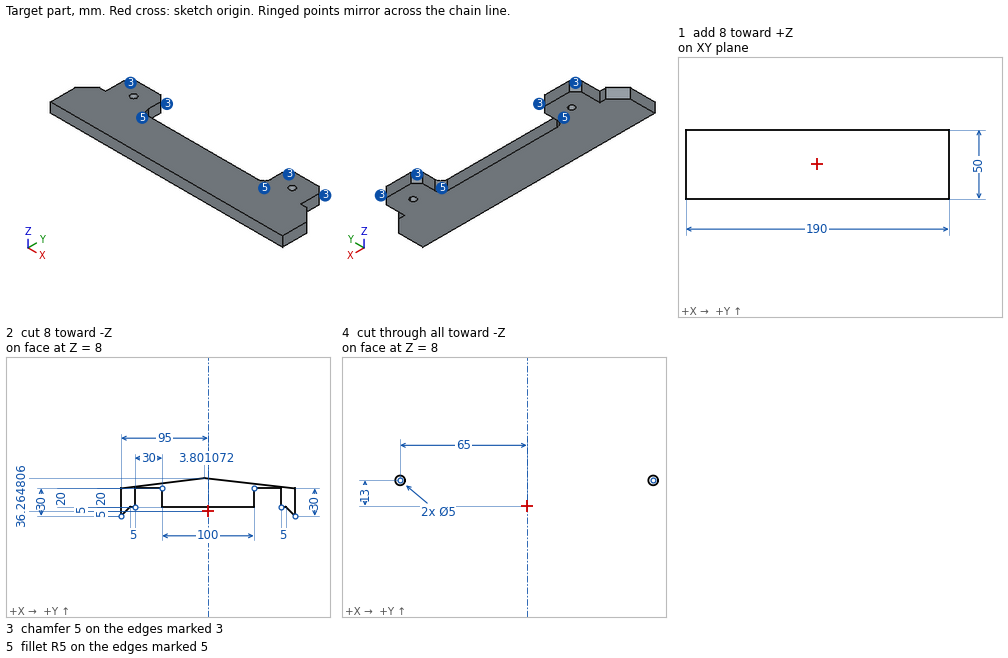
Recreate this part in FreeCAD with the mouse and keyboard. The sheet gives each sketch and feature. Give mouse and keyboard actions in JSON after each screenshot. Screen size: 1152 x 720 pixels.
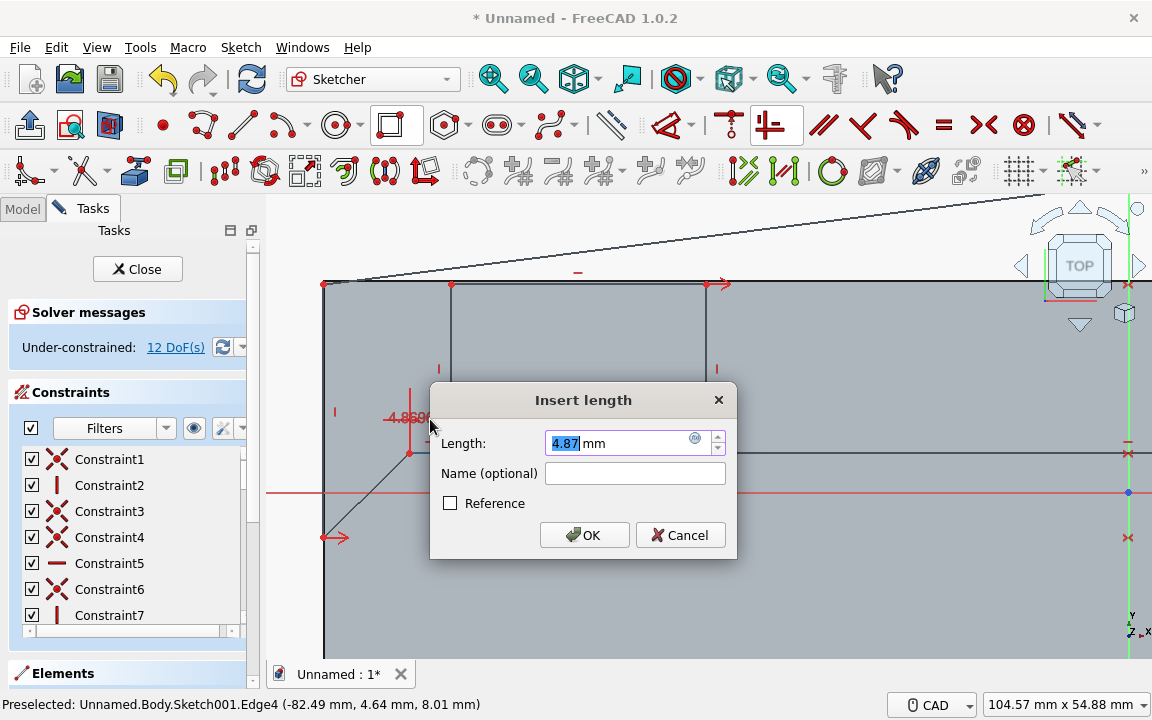
{"action": "type", "text": "5"}
{"action": "key", "text": "Return"}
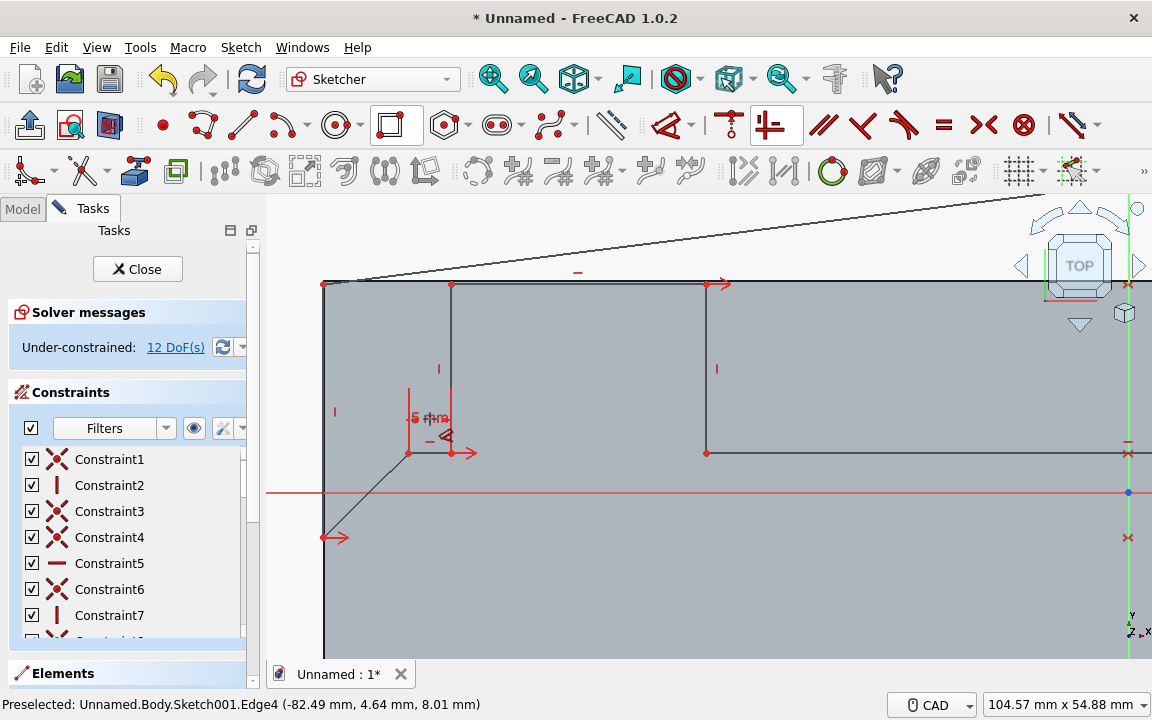
{"action": "scroll", "coordinate": [430, 455], "scroll_direction": "down", "scroll_amount": 6}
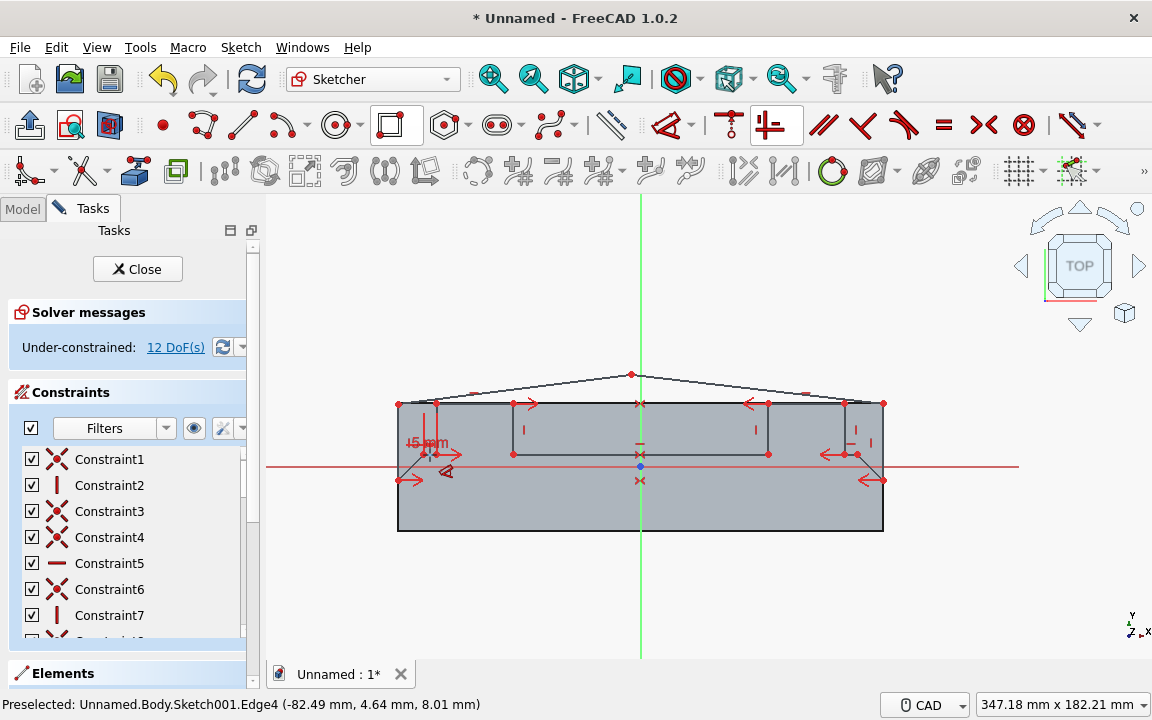
{"action": "scroll", "coordinate": [849, 455], "scroll_direction": "up", "scroll_amount": 7}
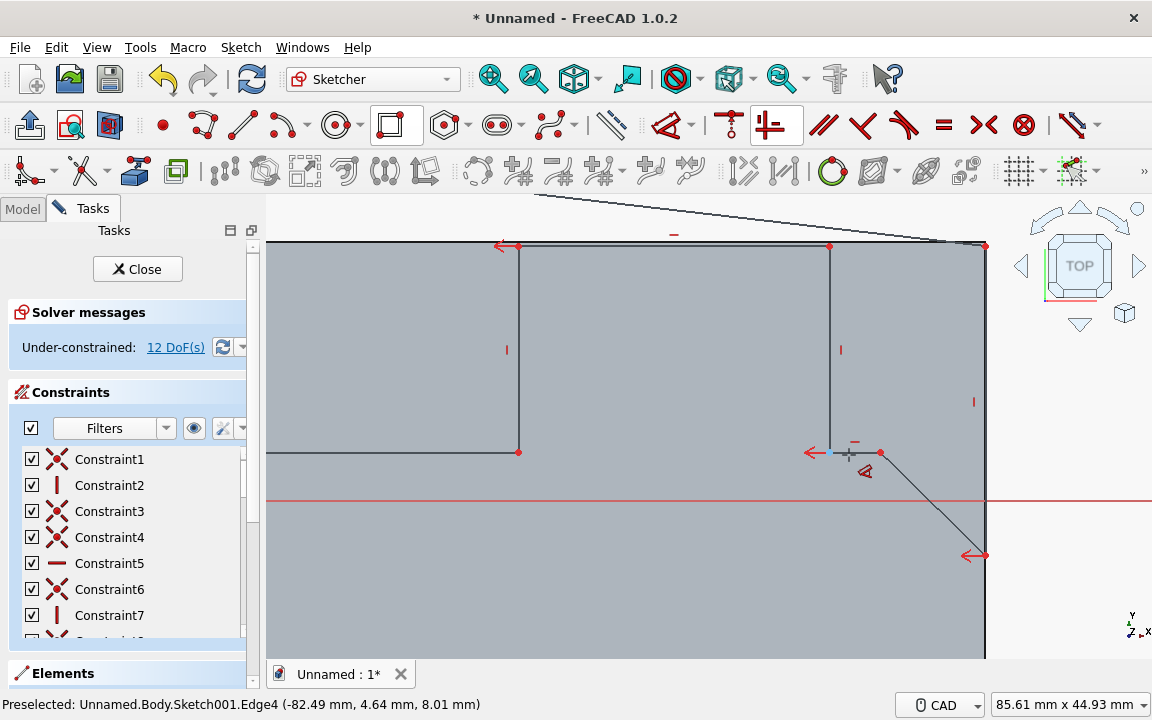
{"action": "left_click", "coordinate": [845, 453]}
{"action": "left_click", "coordinate": [855, 487]}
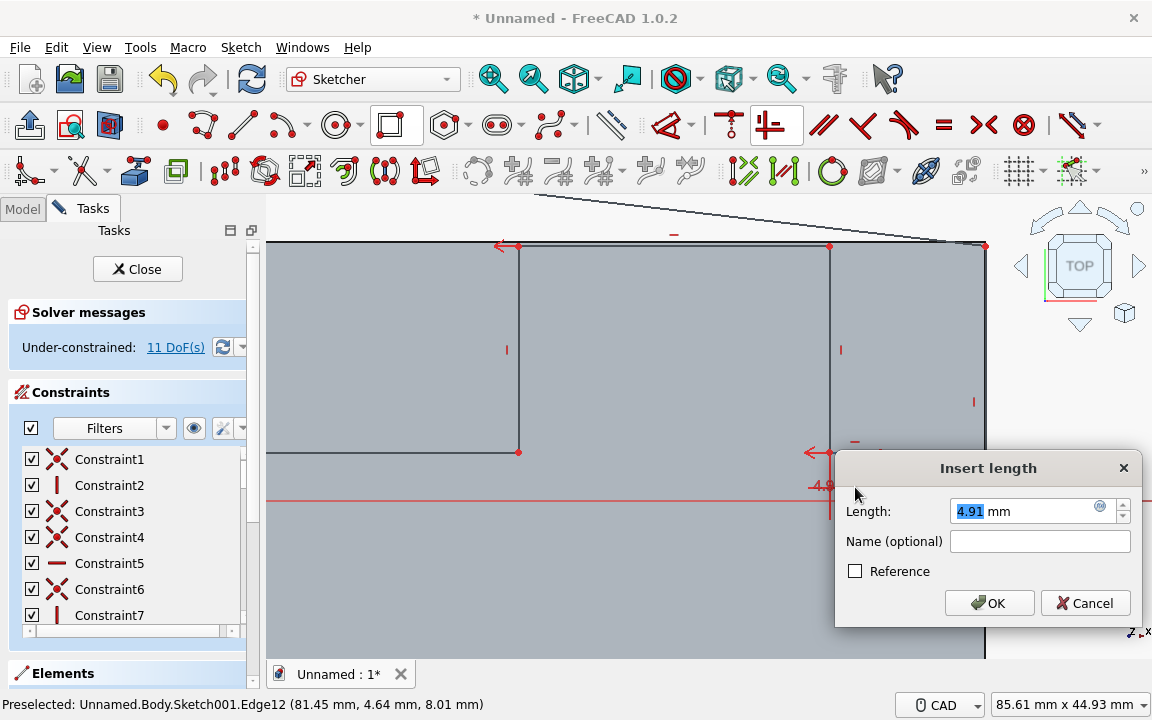
{"action": "type", "text": "5"}
{"action": "key", "text": "Return"}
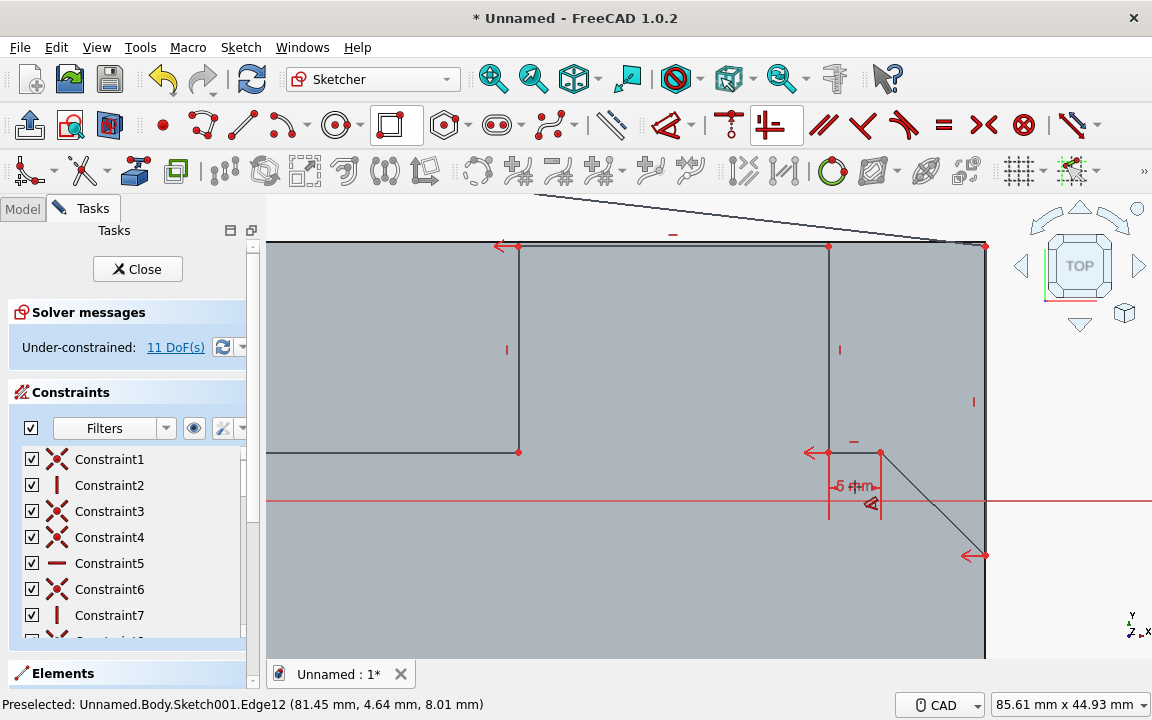
{"action": "scroll", "coordinate": [849, 455], "scroll_direction": "down", "scroll_amount": 7}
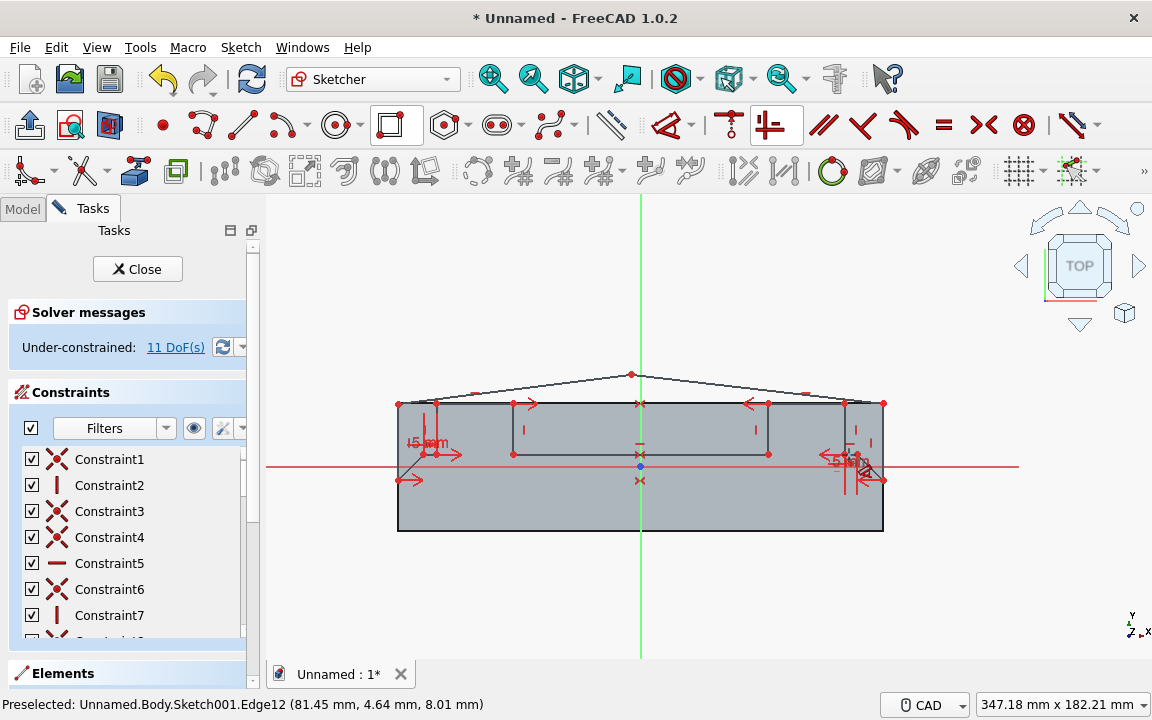
{"action": "left_click", "coordinate": [398, 427]}
{"action": "left_click", "coordinate": [364, 416]}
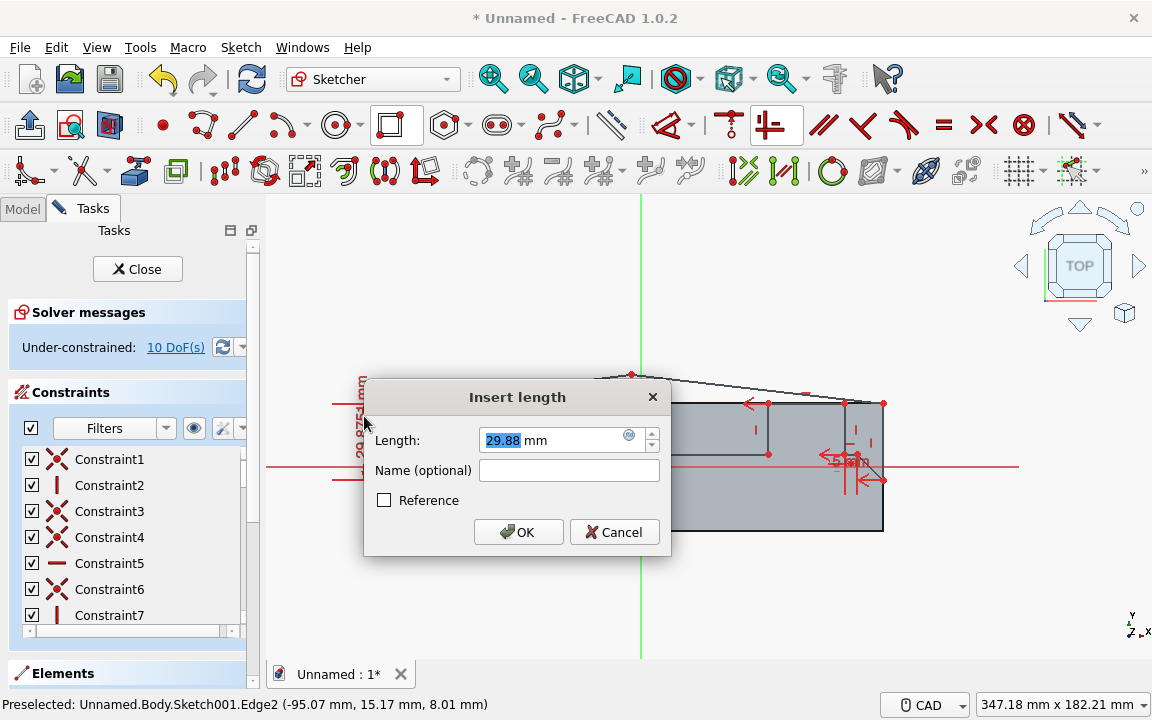
{"action": "type", "text": "30"}
{"action": "key", "text": "Return"}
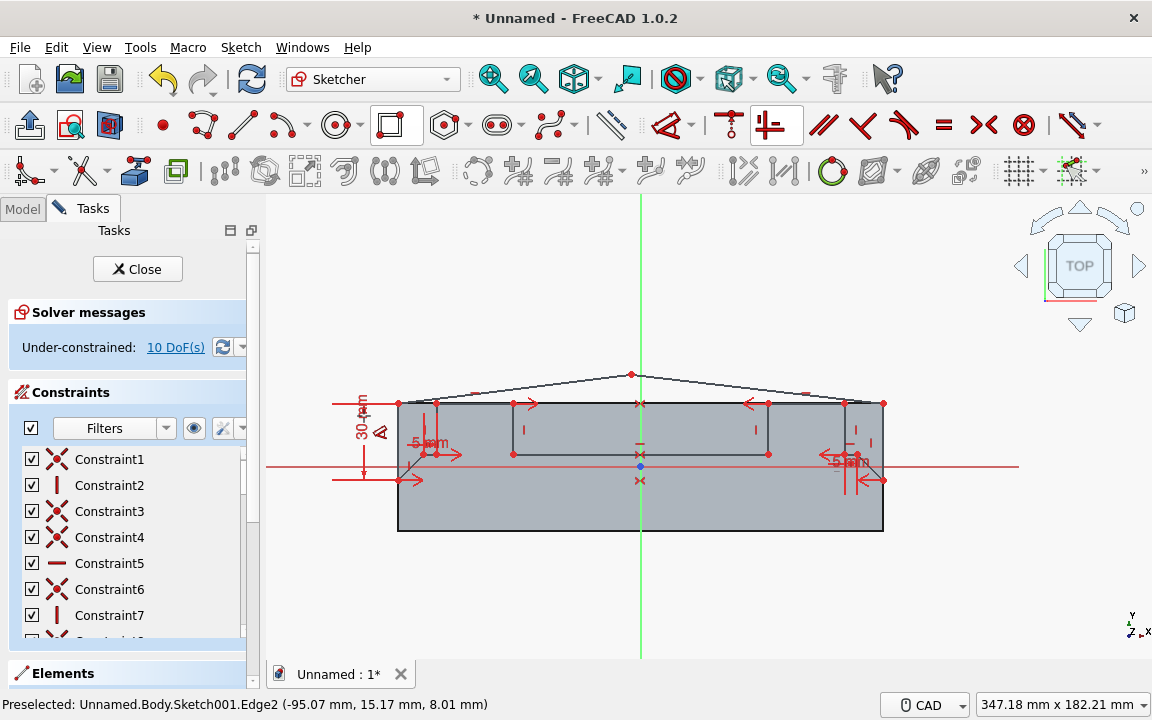
{"action": "left_click", "coordinate": [437, 440]}
{"action": "left_click", "coordinate": [471, 418]}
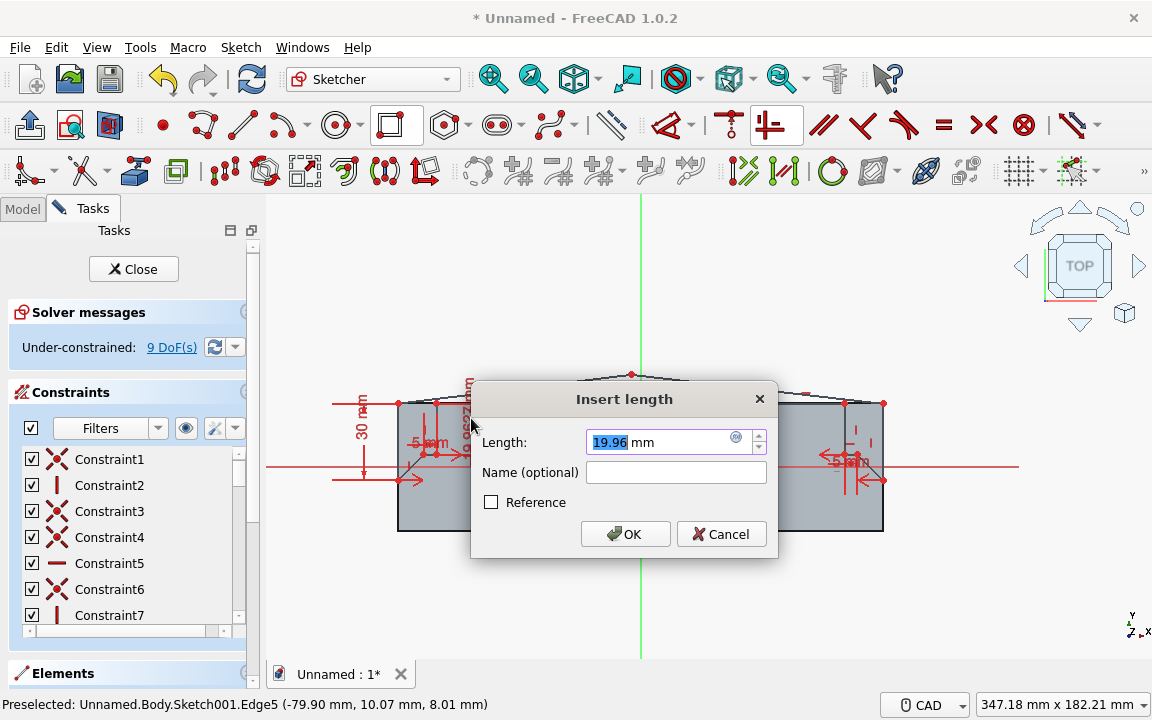
{"action": "type", "text": "20"}
{"action": "key", "text": "Return"}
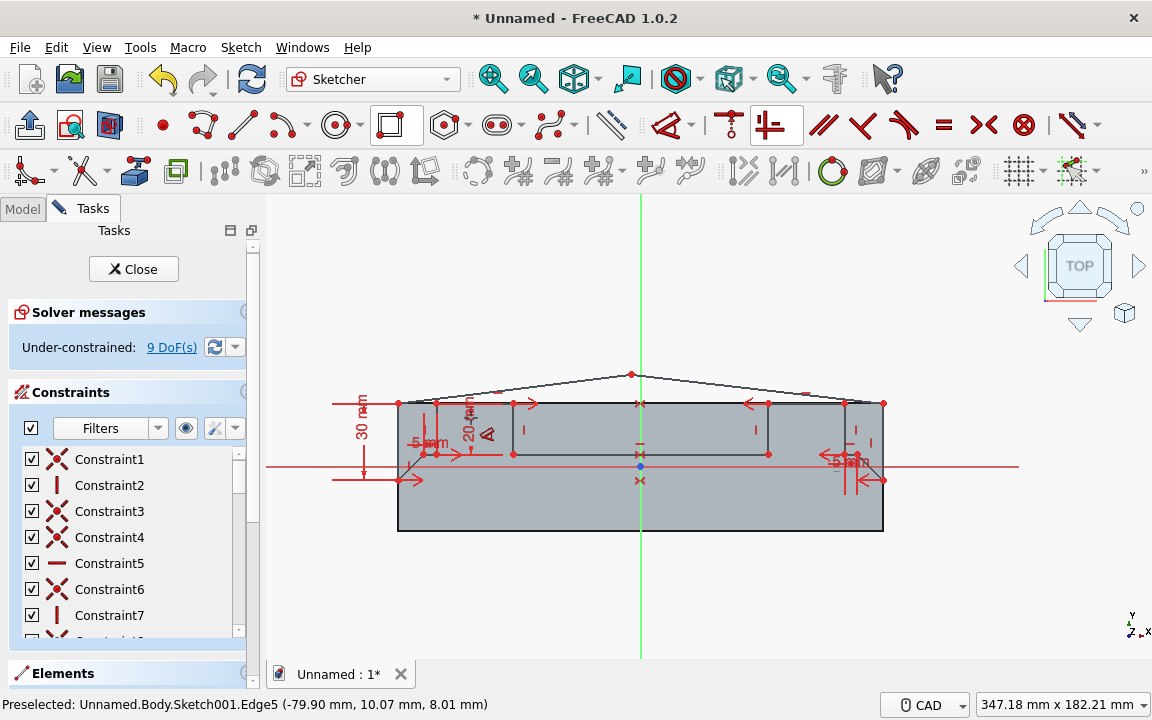
{"action": "left_click", "coordinate": [490, 404]}
{"action": "left_click", "coordinate": [475, 370]}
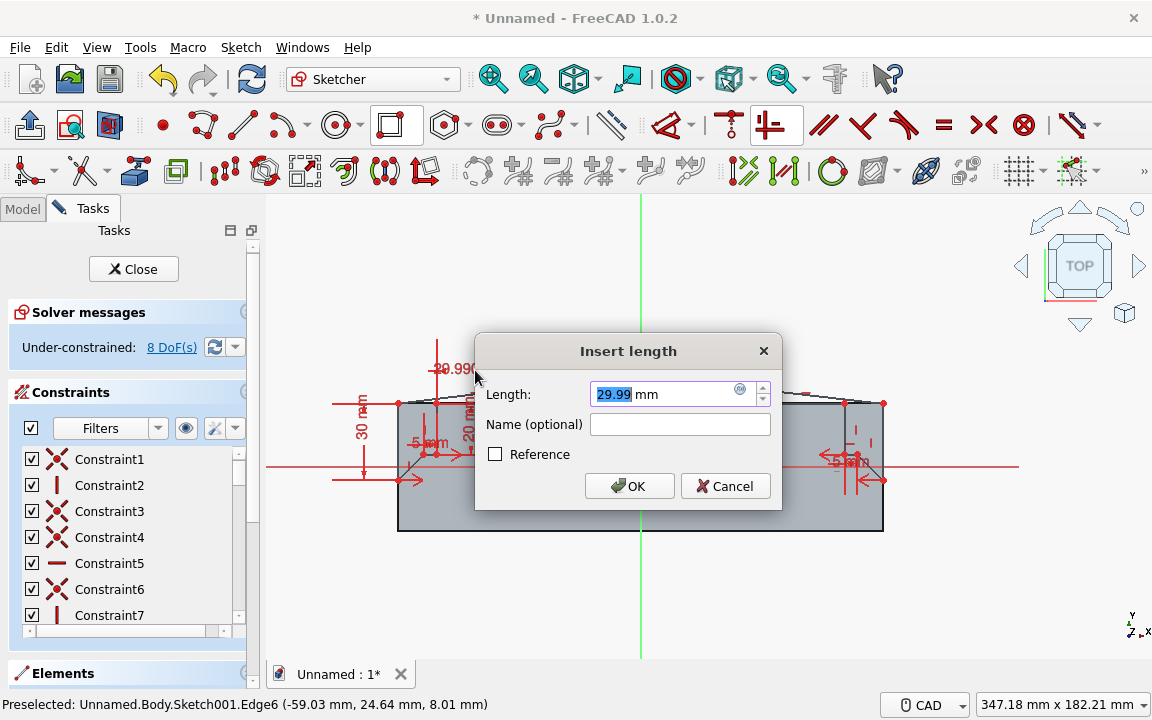
{"action": "type", "text": "30"}
{"action": "key", "text": "Return"}